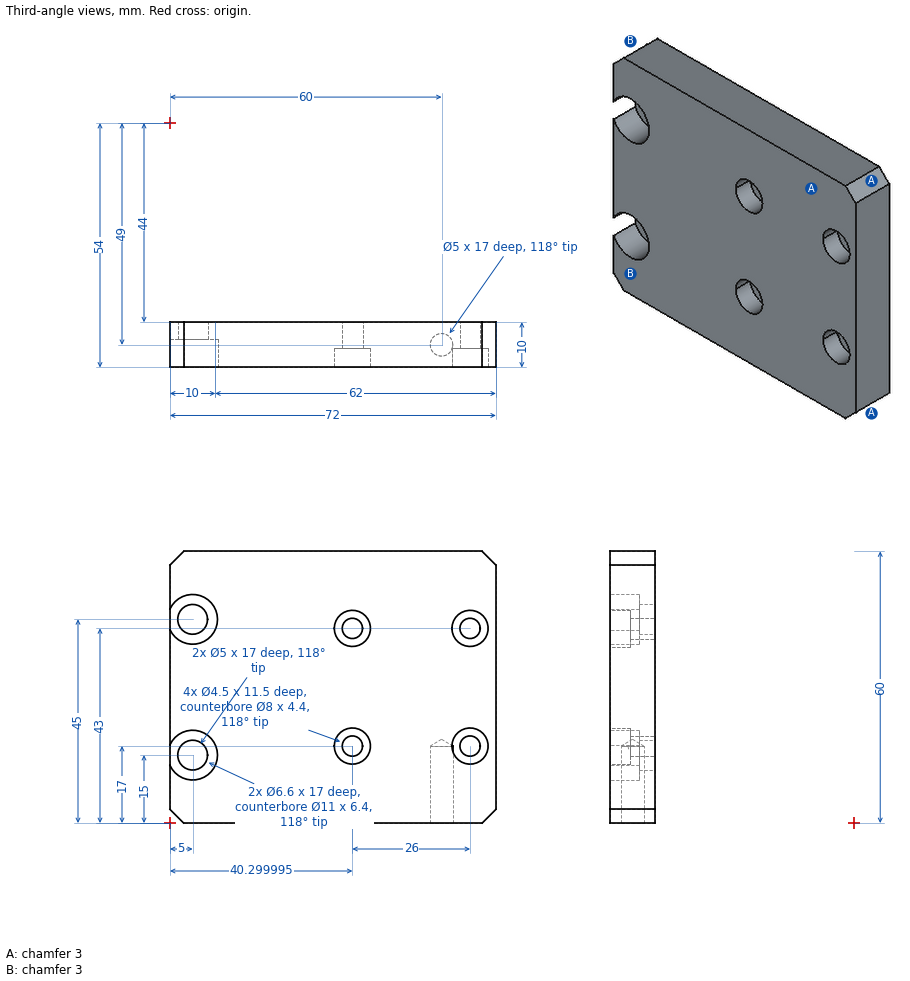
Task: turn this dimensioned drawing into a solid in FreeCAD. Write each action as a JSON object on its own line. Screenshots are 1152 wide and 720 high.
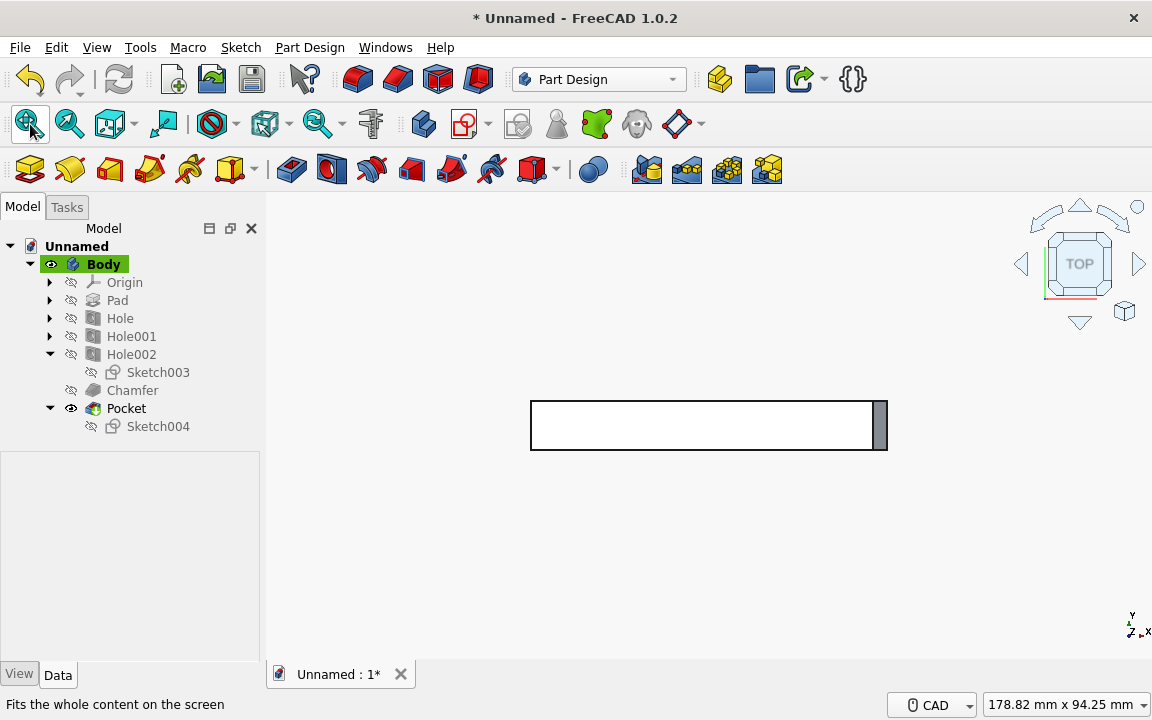
{"action": "left_click", "coordinate": [531, 424]}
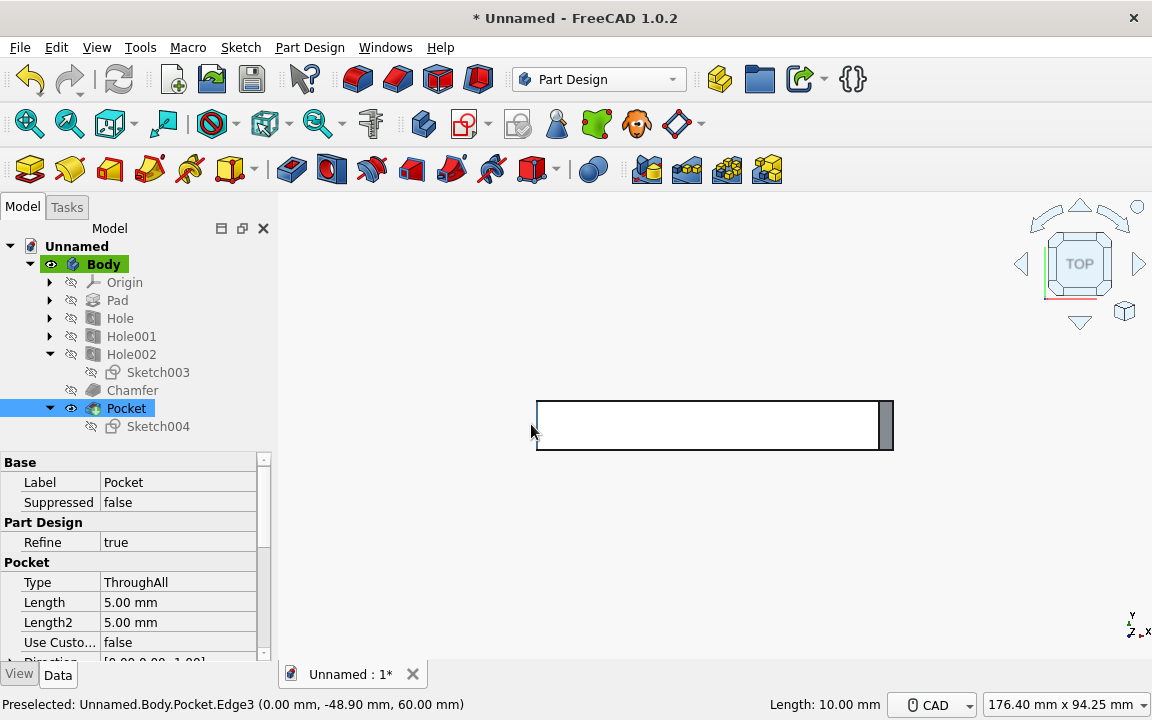
{"action": "key", "text": "0"}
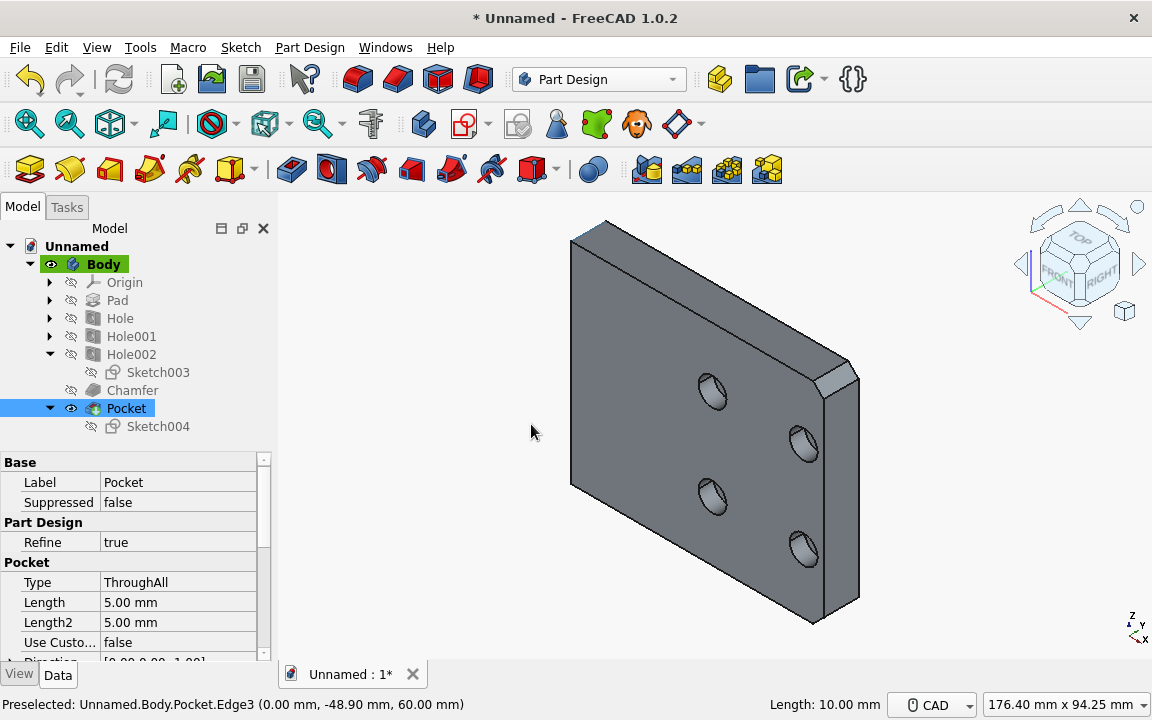
{"action": "key", "text": "1"}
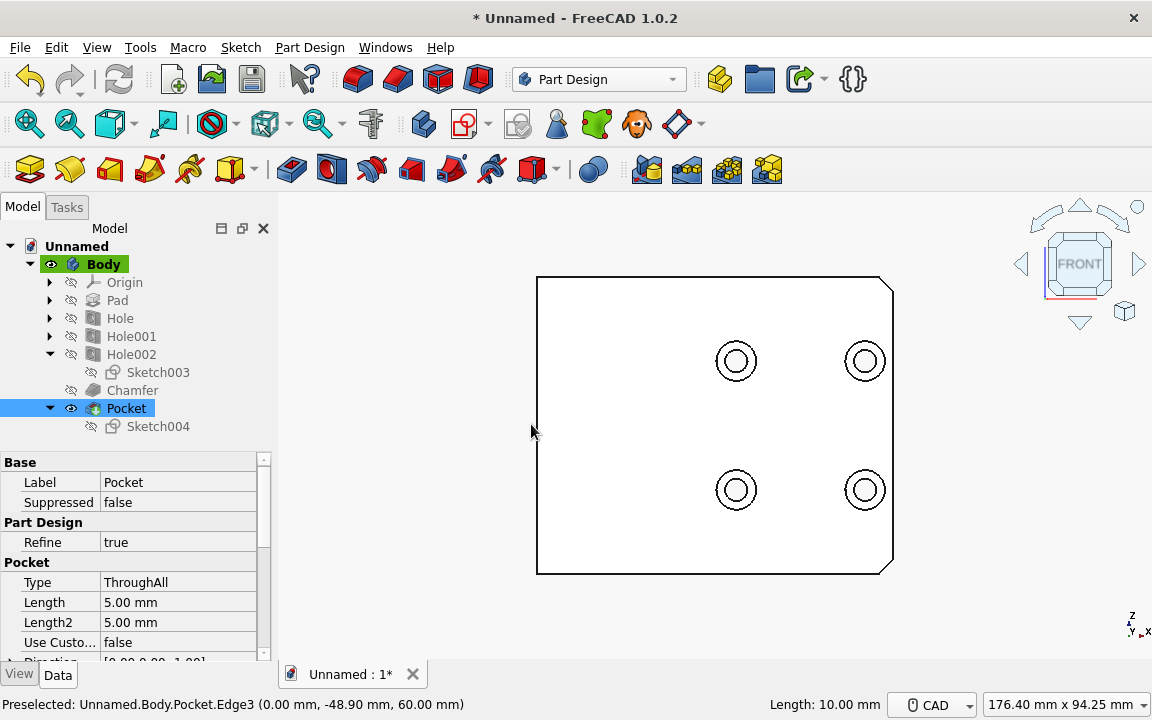
{"action": "key", "text": "3"}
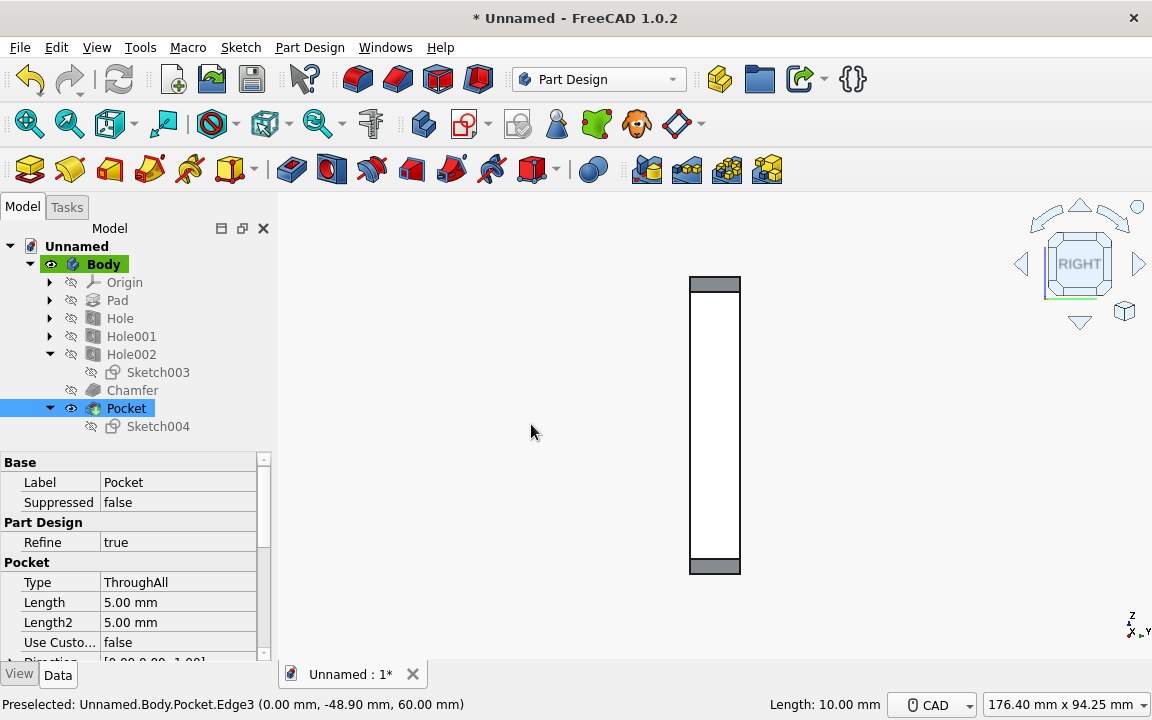
{"action": "key", "text": "5"}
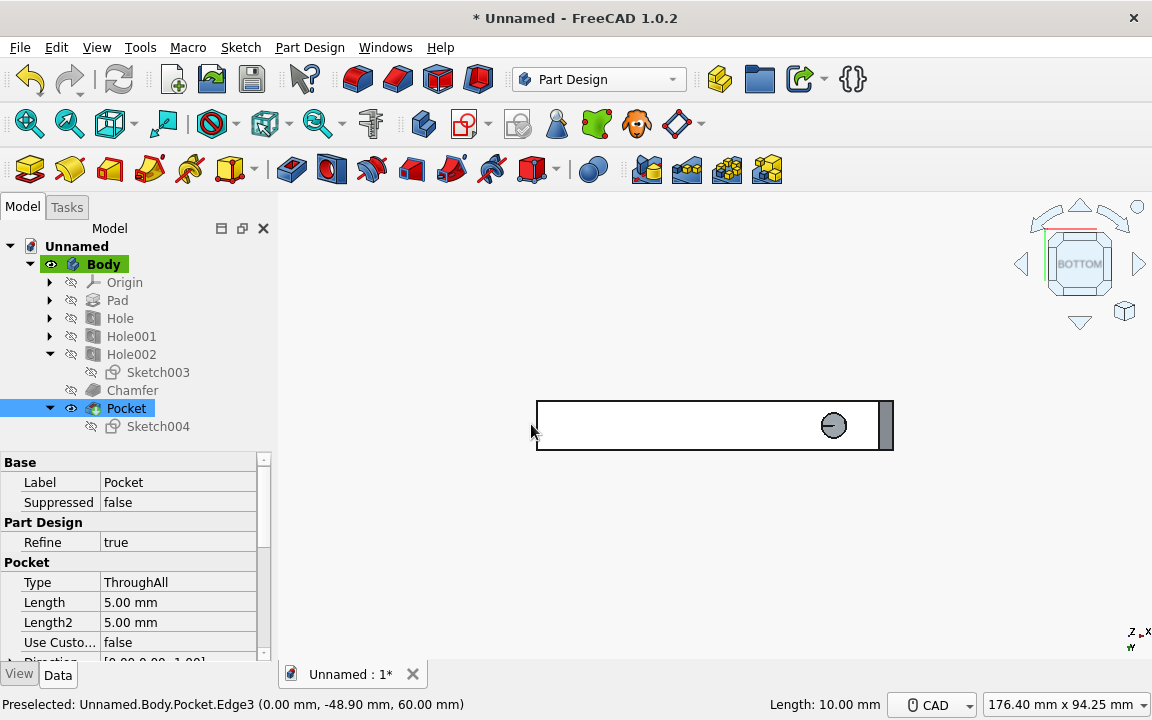
{"action": "left_click", "coordinate": [30, 124]}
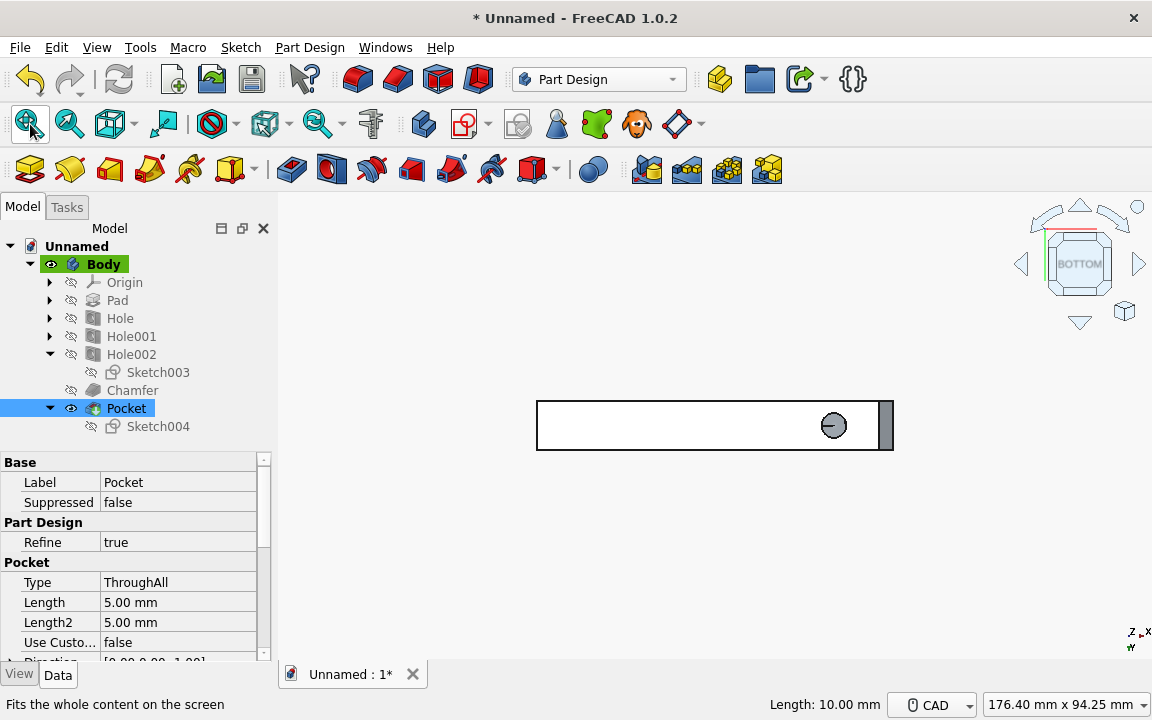
{"action": "left_click", "coordinate": [537, 424], "text": "ctrl"}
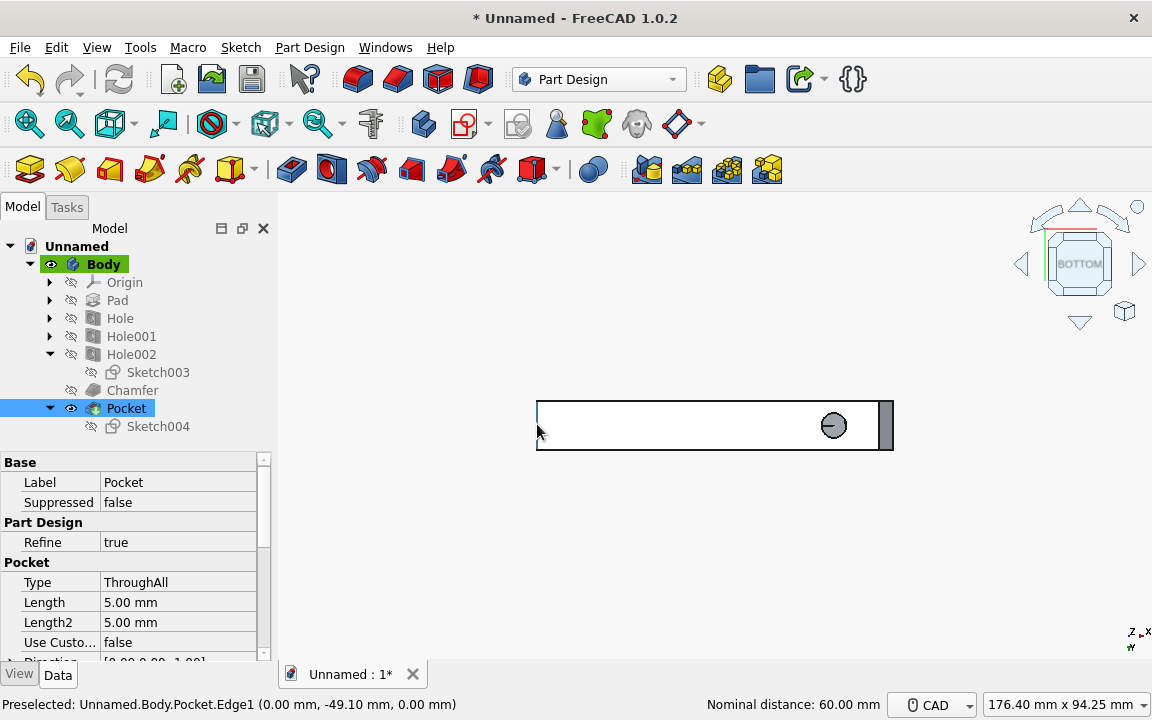
{"action": "left_click", "coordinate": [398, 80]}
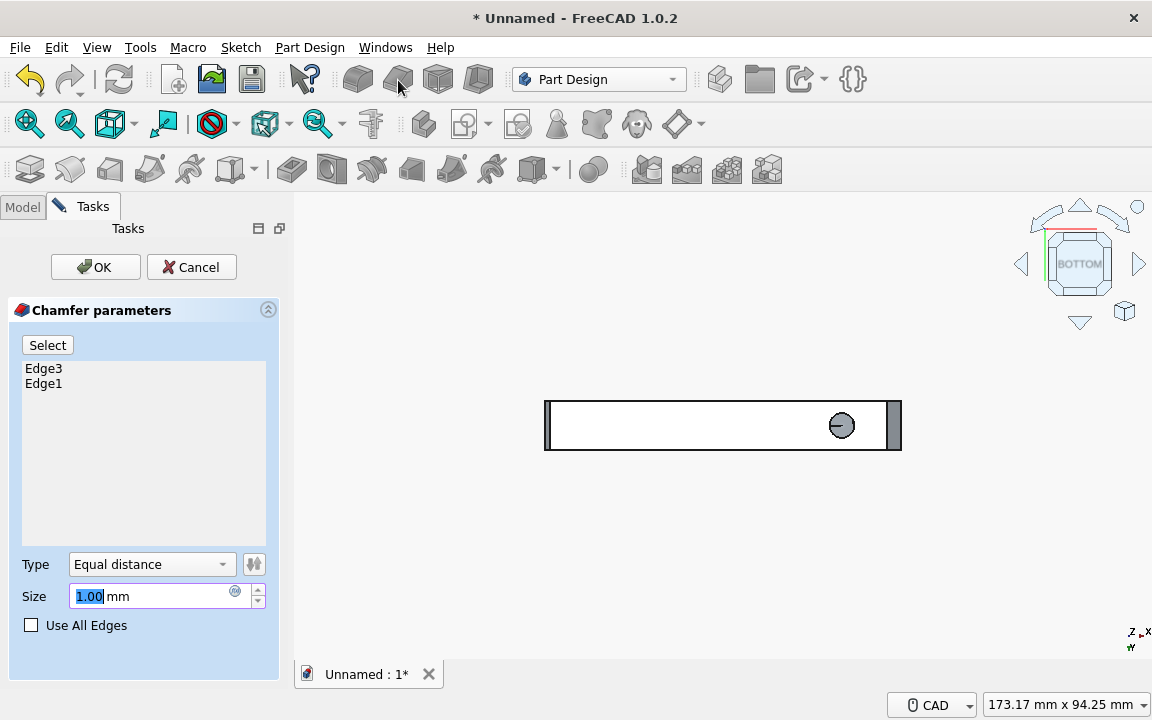
{"action": "type", "text": "3"}
{"action": "key", "text": "Tab"}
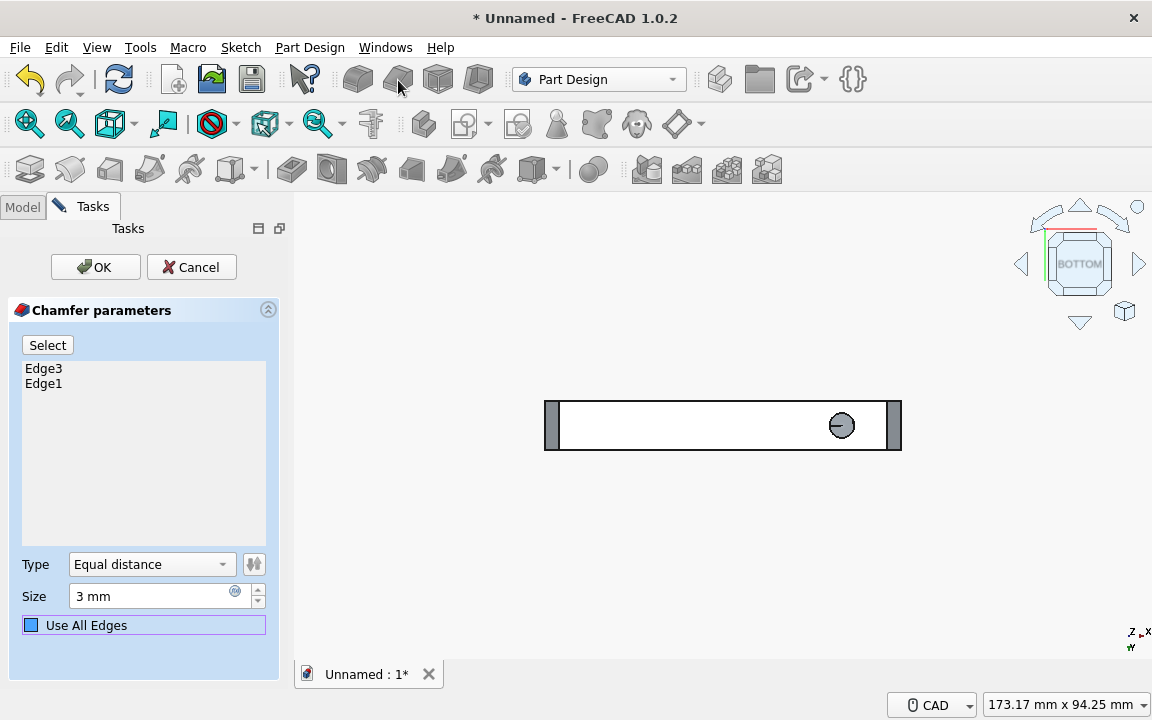
{"action": "left_click", "coordinate": [96, 267]}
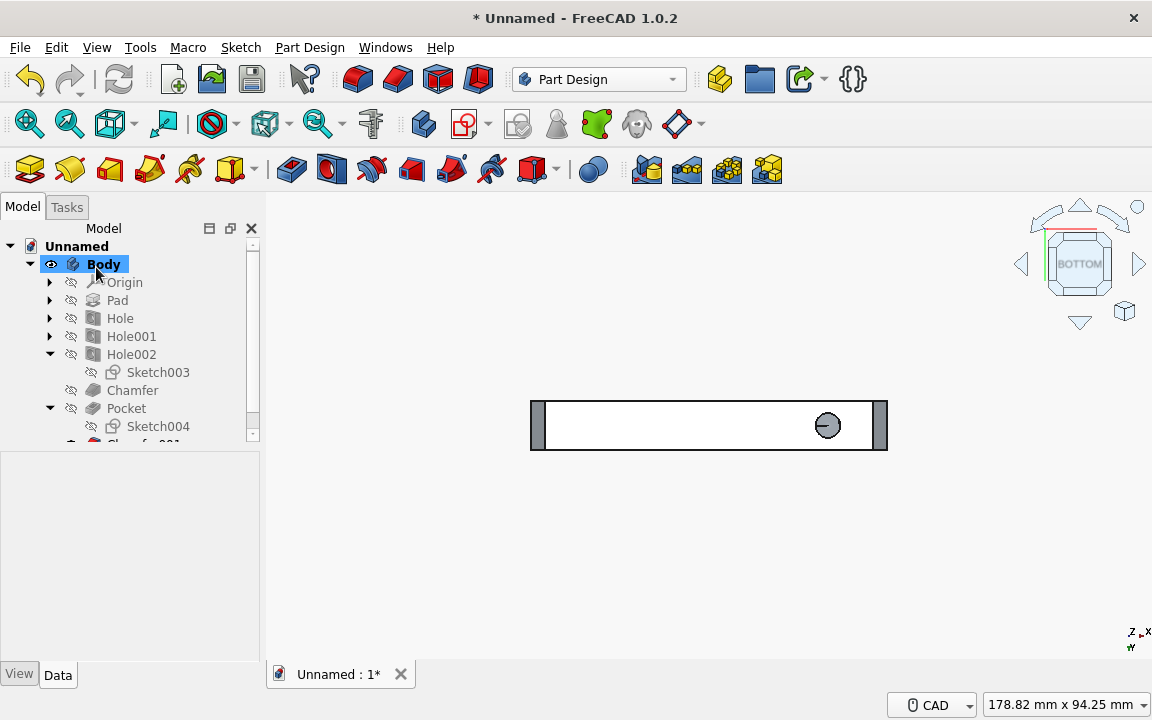
{"action": "left_click", "coordinate": [30, 124]}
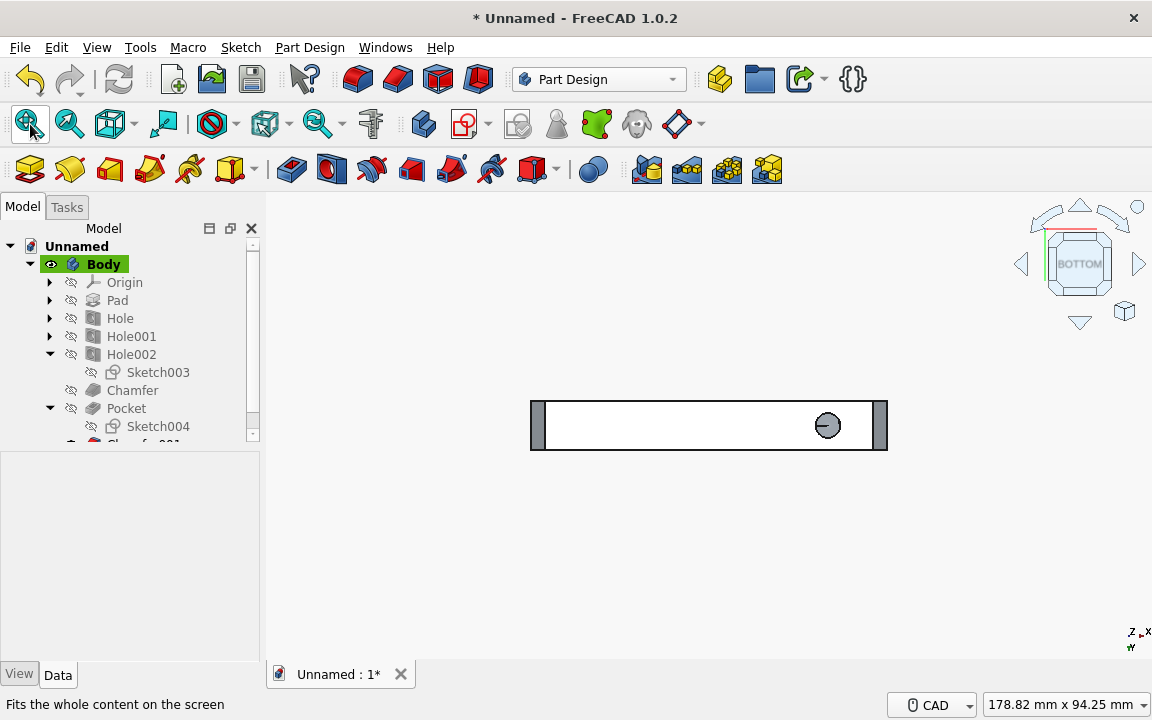
{"action": "key", "text": "0"}